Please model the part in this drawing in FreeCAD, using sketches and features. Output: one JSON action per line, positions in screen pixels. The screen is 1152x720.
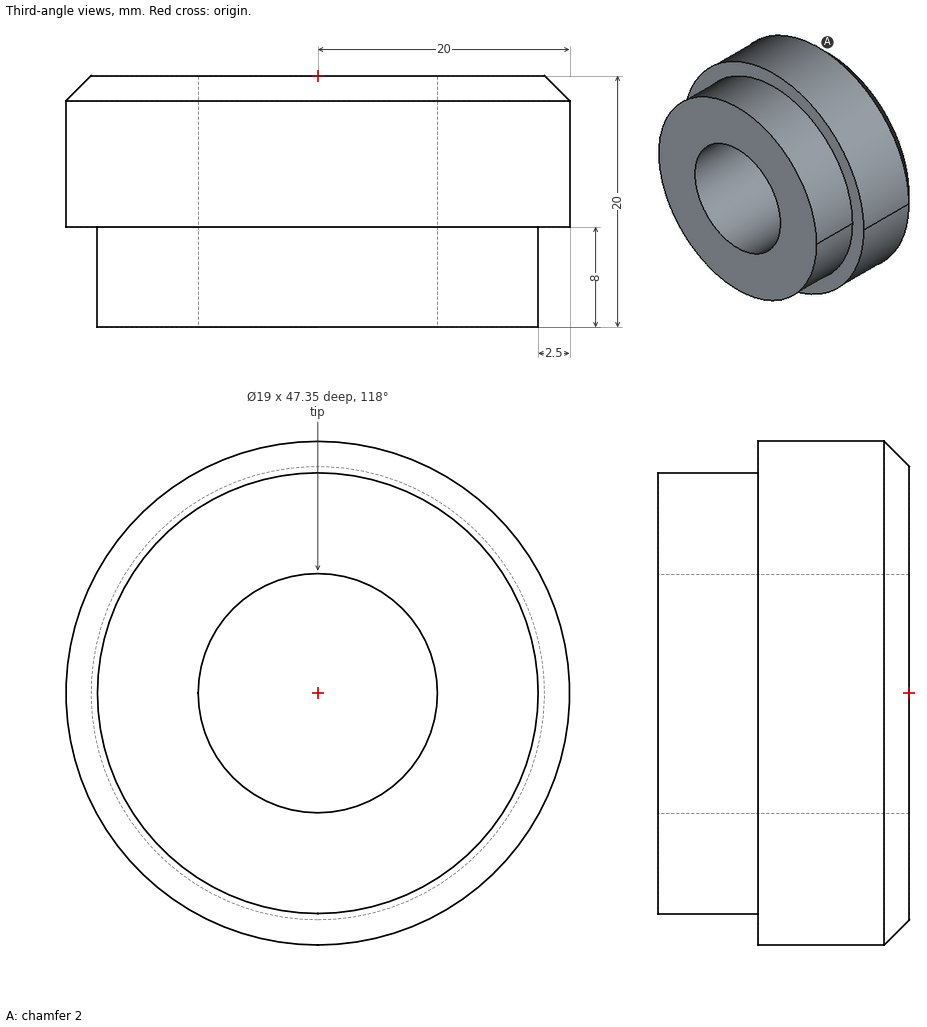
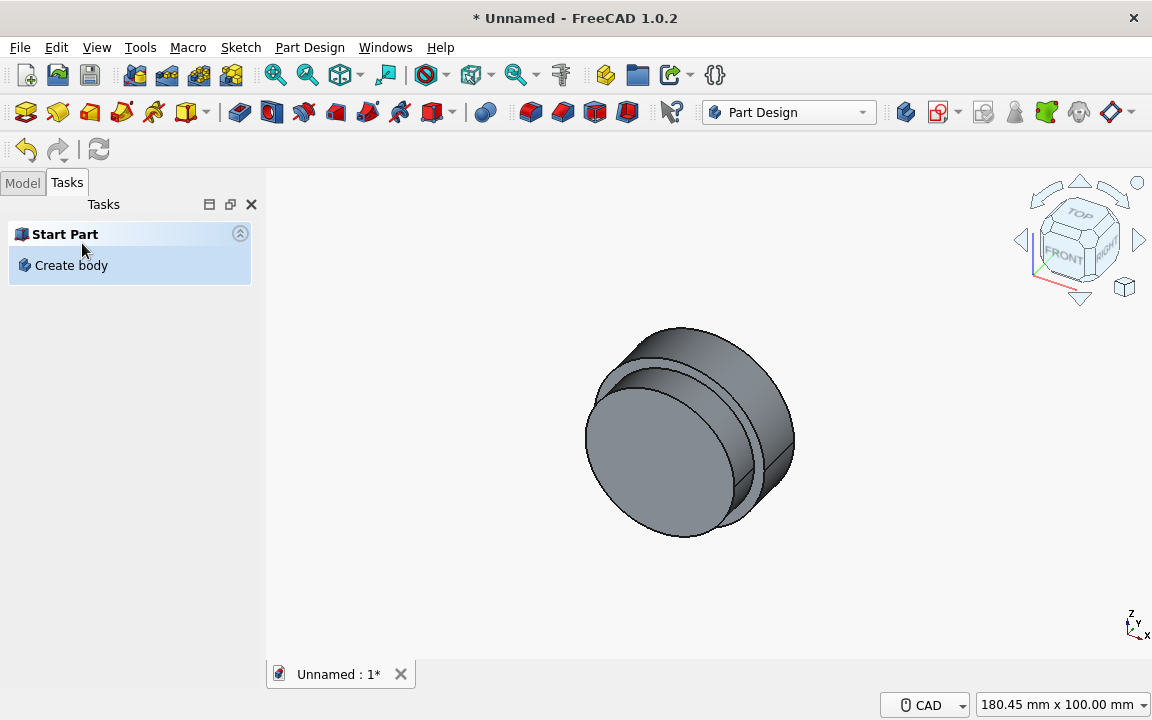
{"action": "key", "text": "4"}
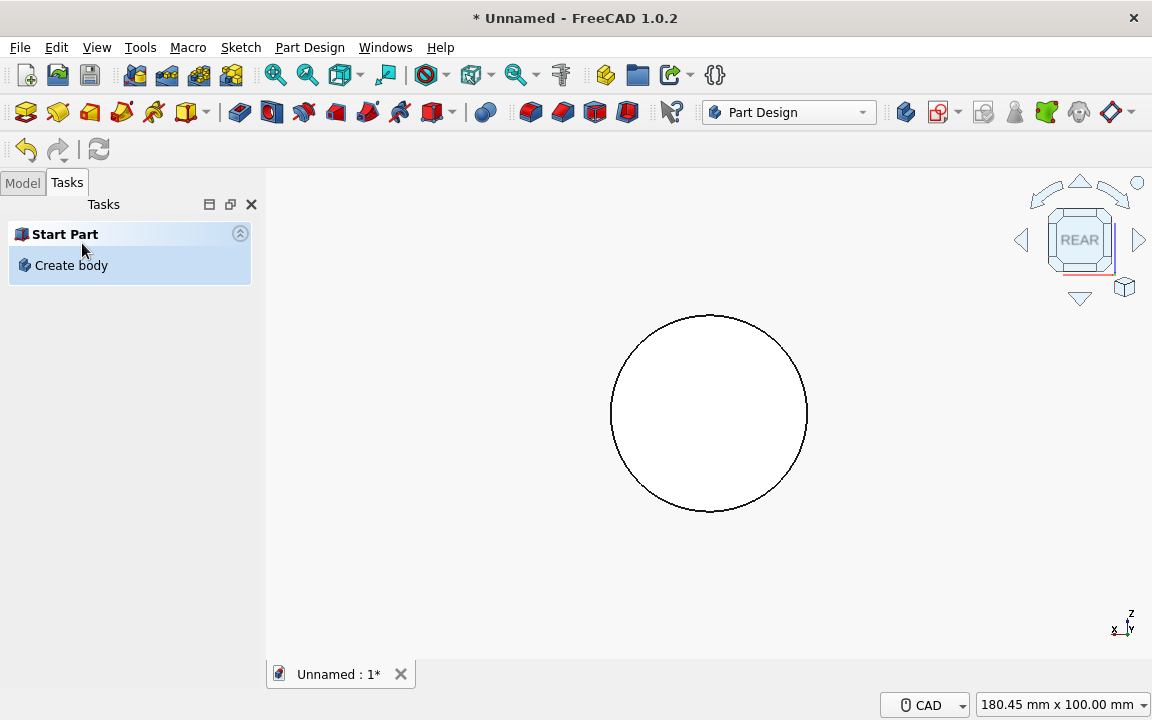
{"action": "left_click", "coordinate": [276, 76]}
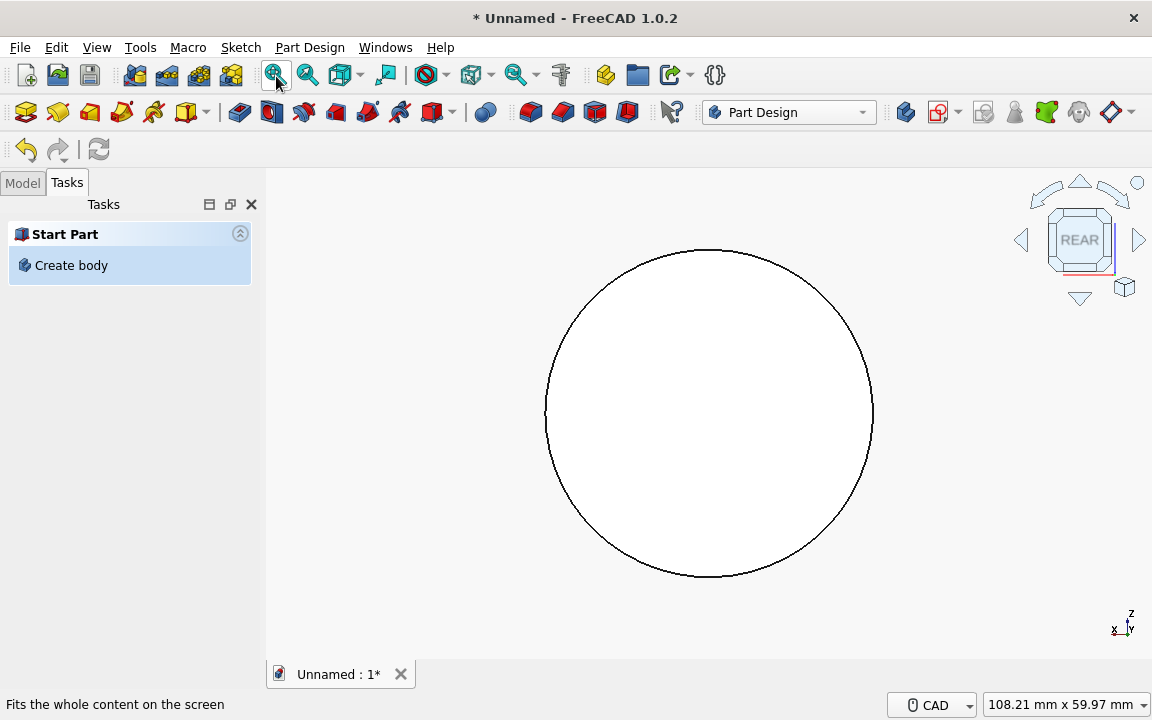
{"action": "left_click", "coordinate": [709, 413]}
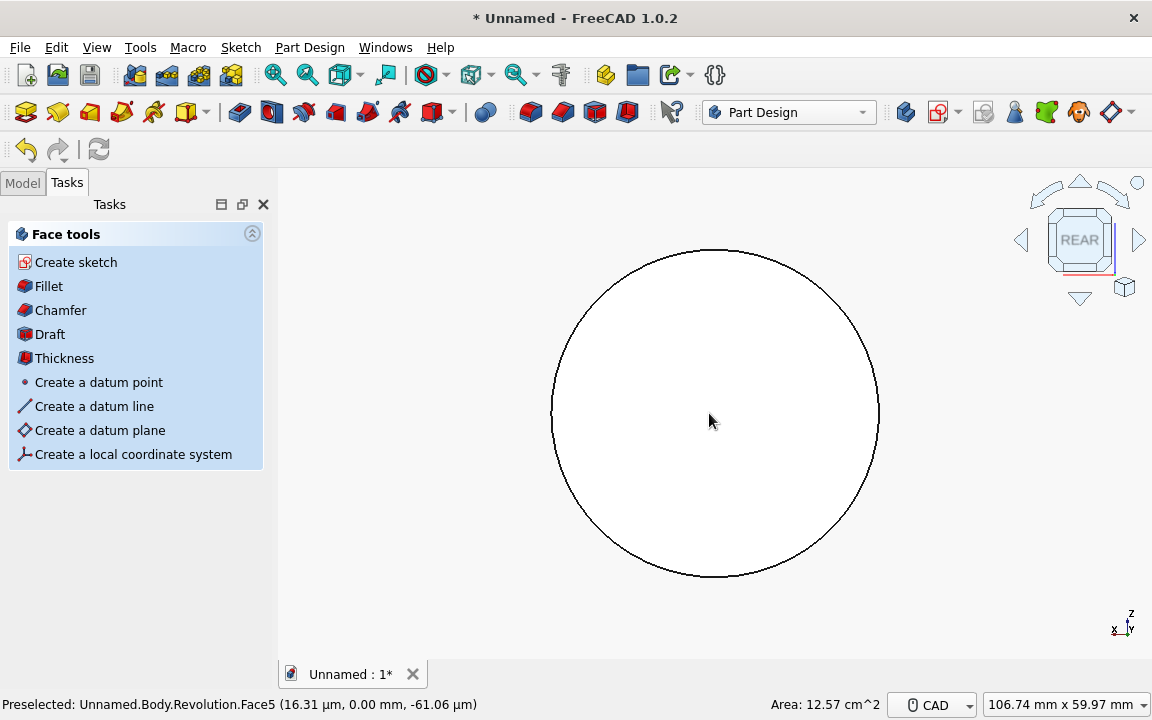
{"action": "left_click", "coordinate": [938, 112]}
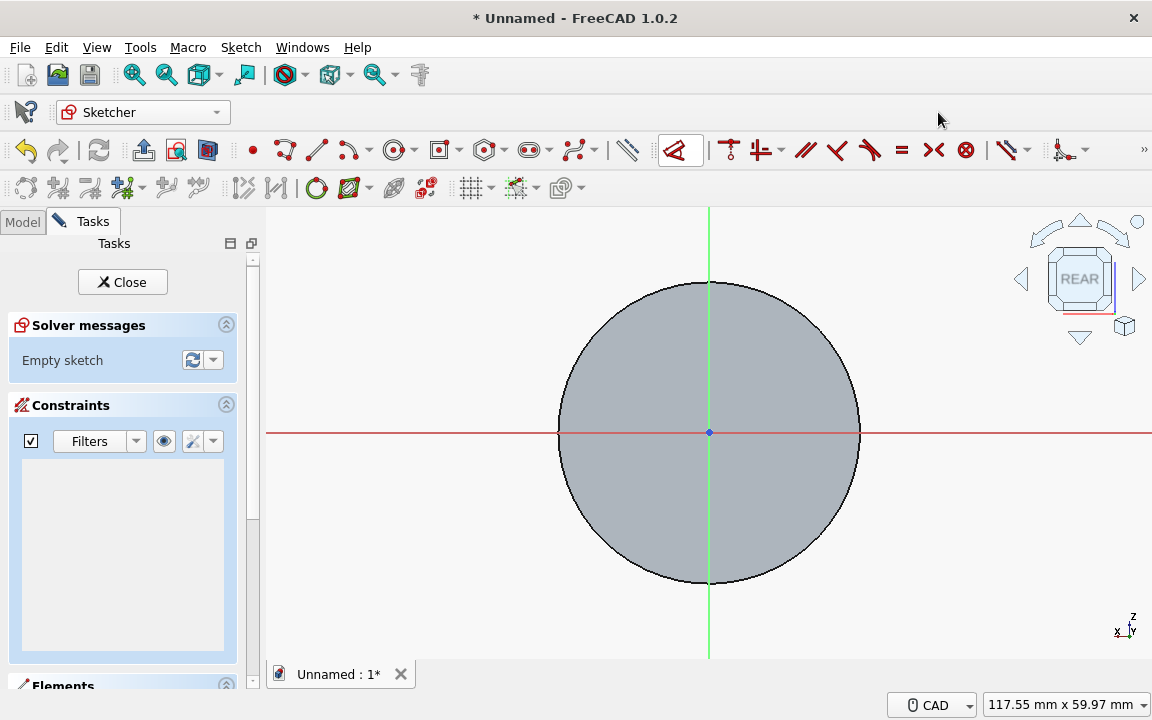
{"action": "scroll", "coordinate": [793, 433], "scroll_direction": "up", "scroll_amount": 3}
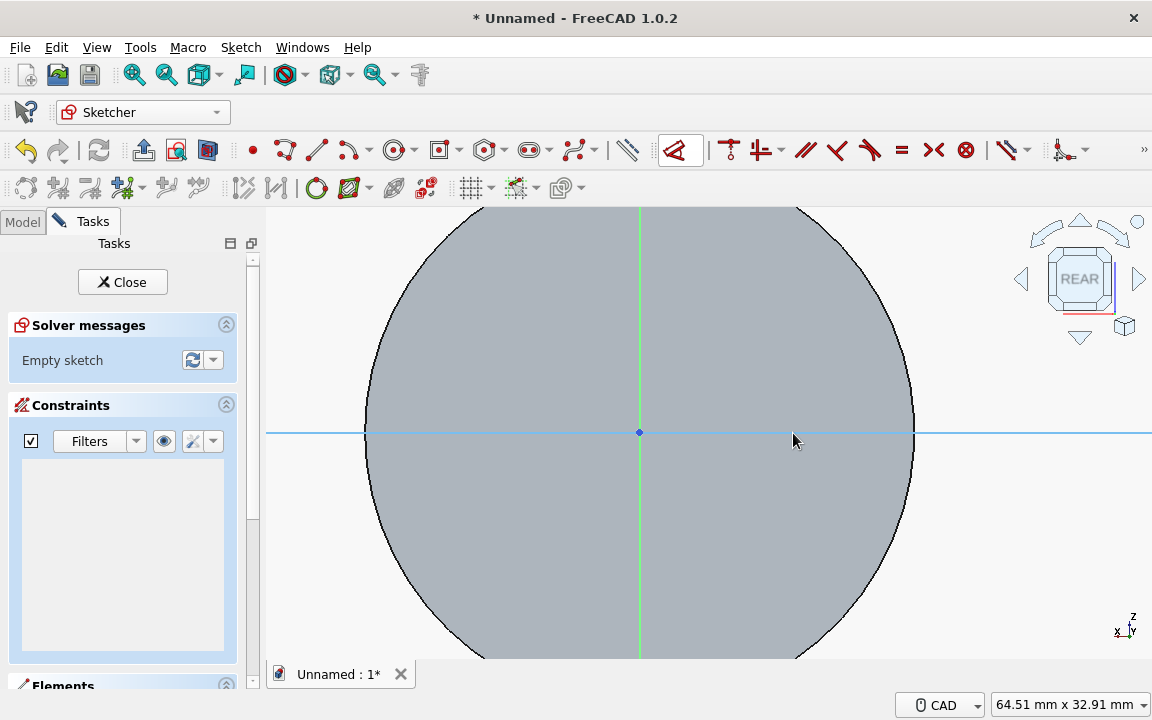
{"action": "left_click", "coordinate": [394, 150]}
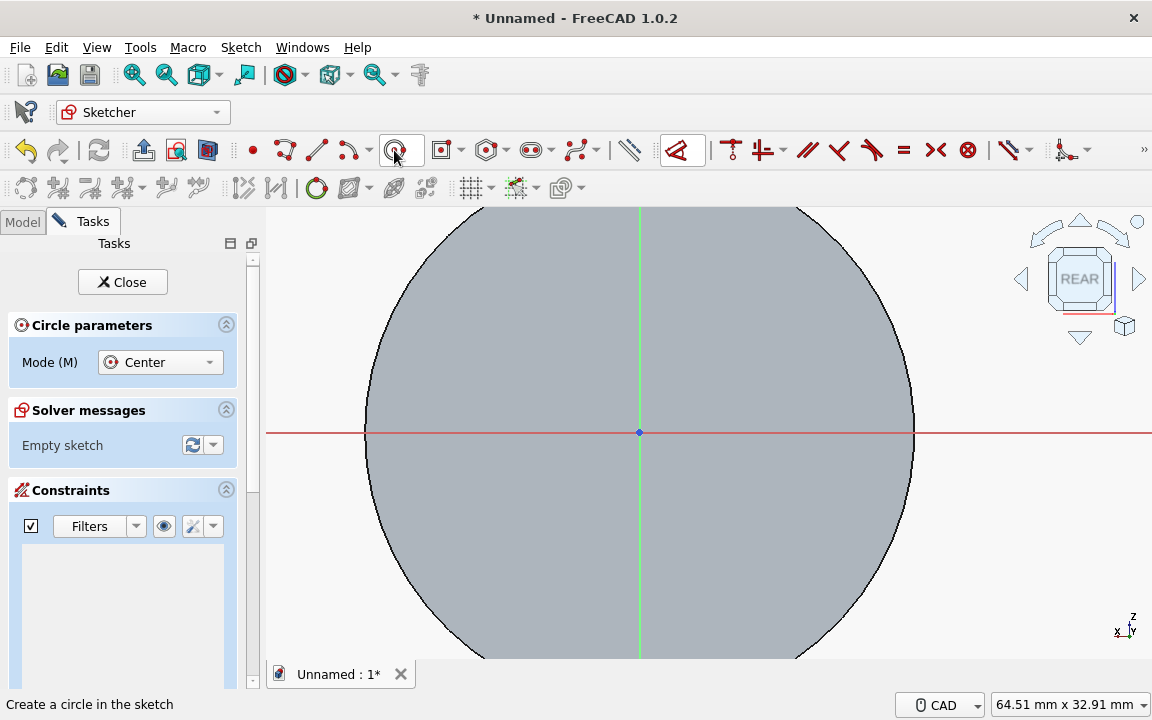
{"action": "left_click", "coordinate": [640, 433]}
{"action": "mouse_move", "coordinate": [732, 340]}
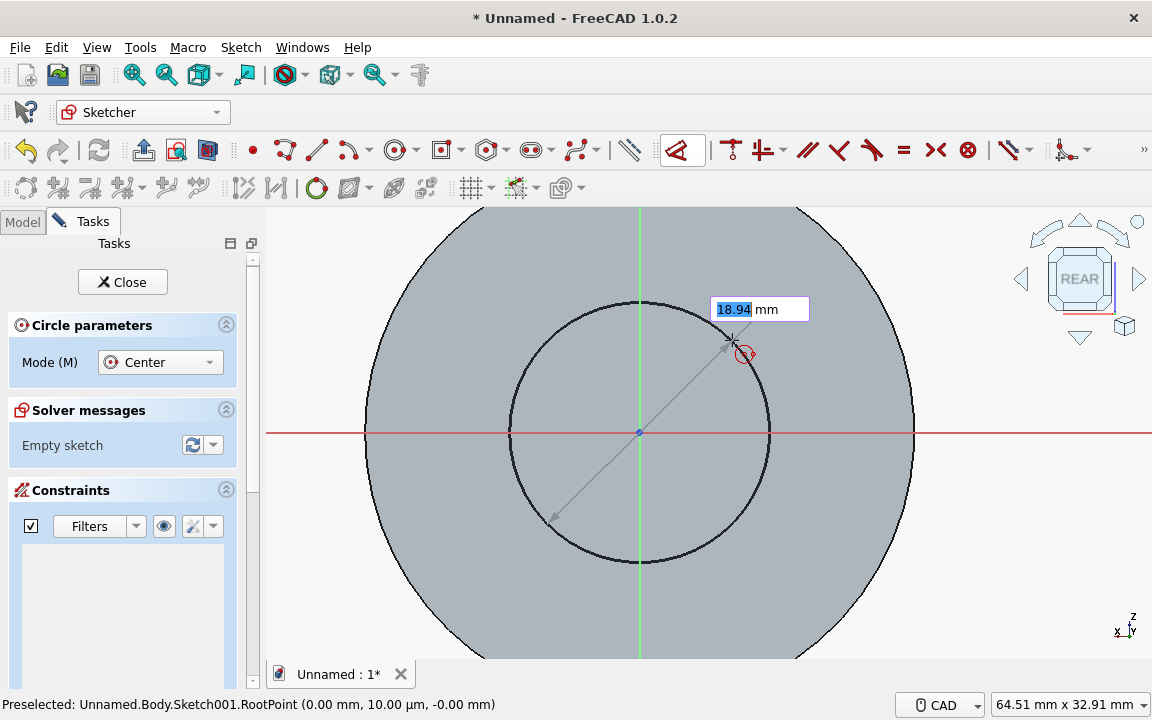
{"action": "type", "text": "19"}
{"action": "key", "text": "Return"}
{"action": "key", "text": "Escape"}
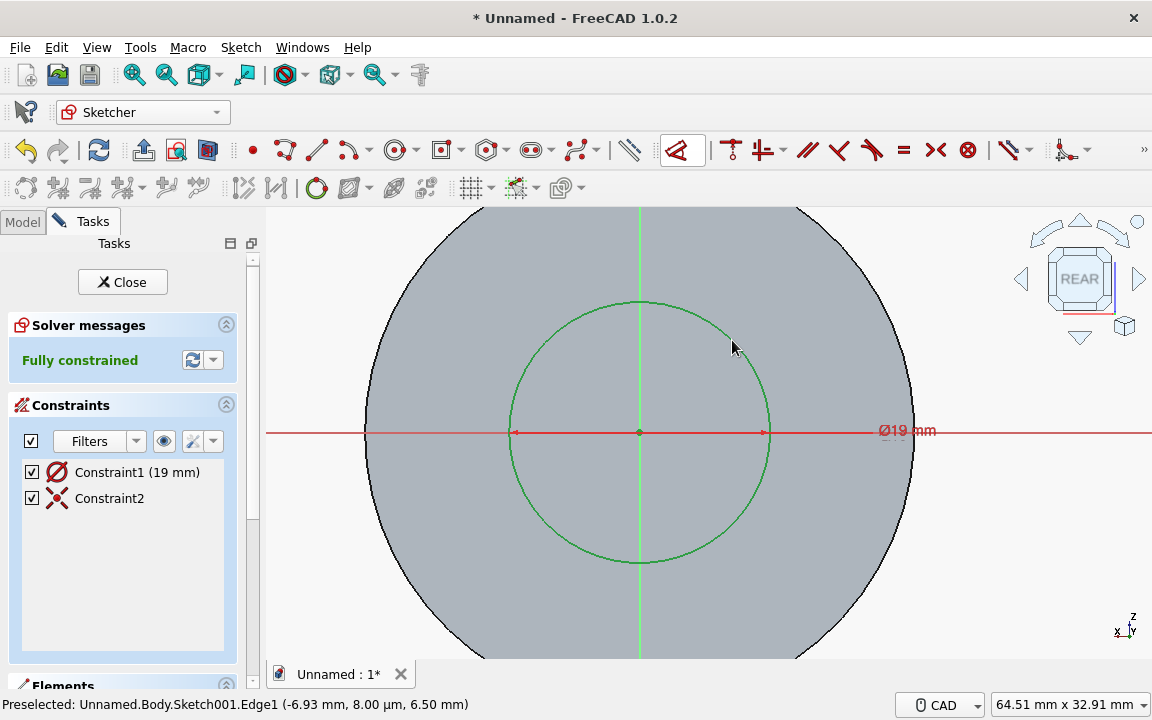
{"action": "left_click", "coordinate": [123, 282]}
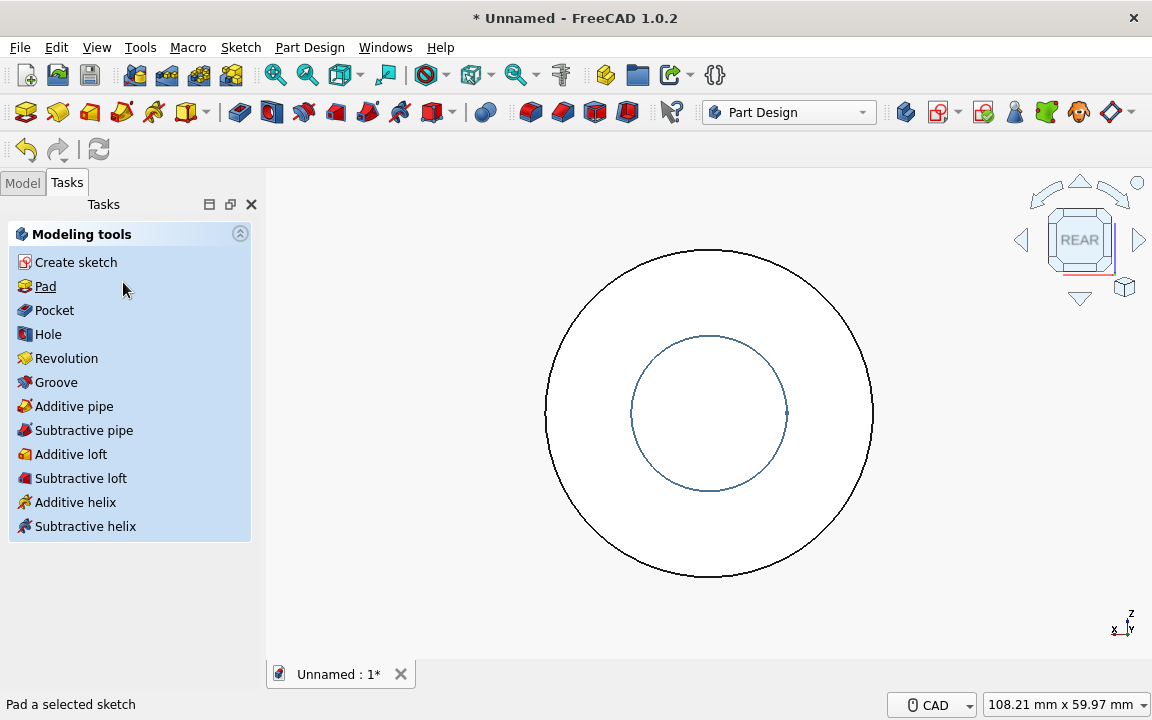
{"action": "left_click", "coordinate": [272, 112]}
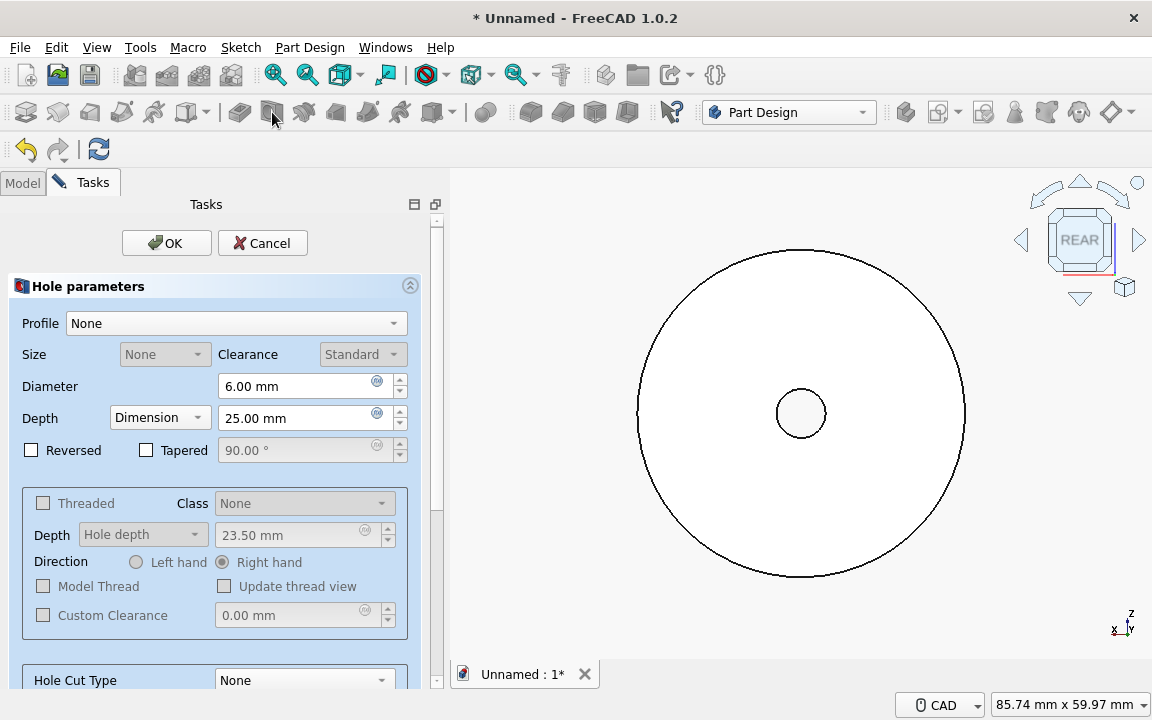
{"action": "triple_click", "coordinate": [305, 386]}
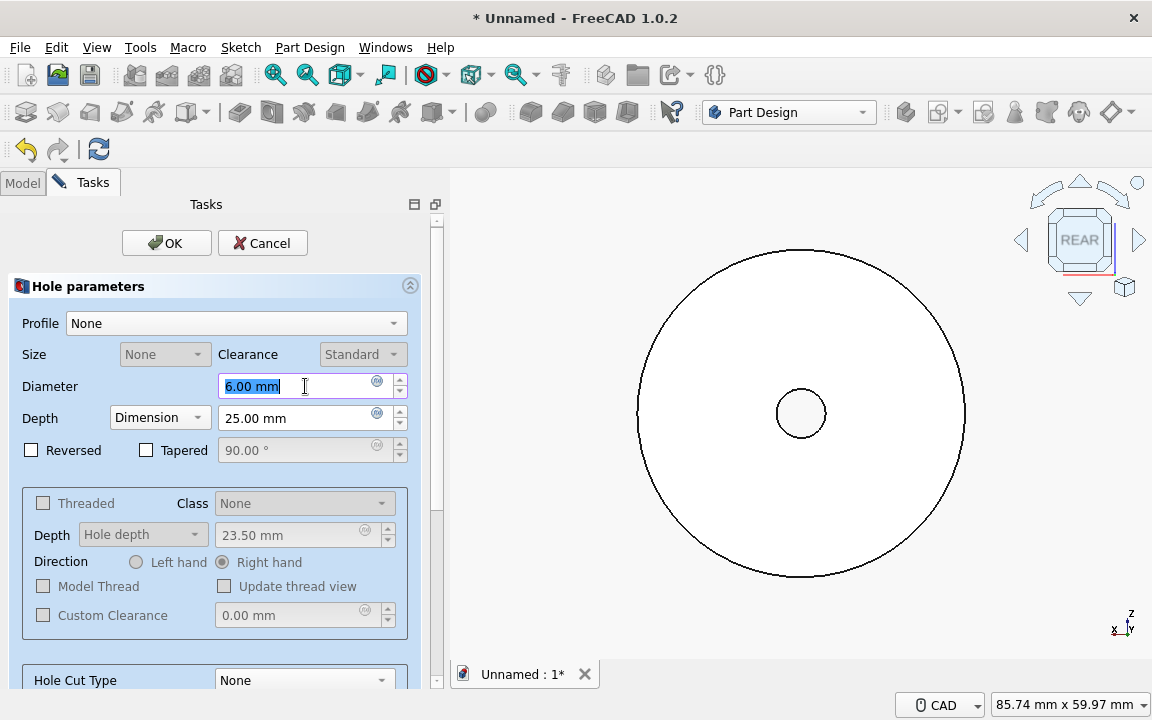
{"action": "type", "text": "19"}
{"action": "key", "text": "Tab"}